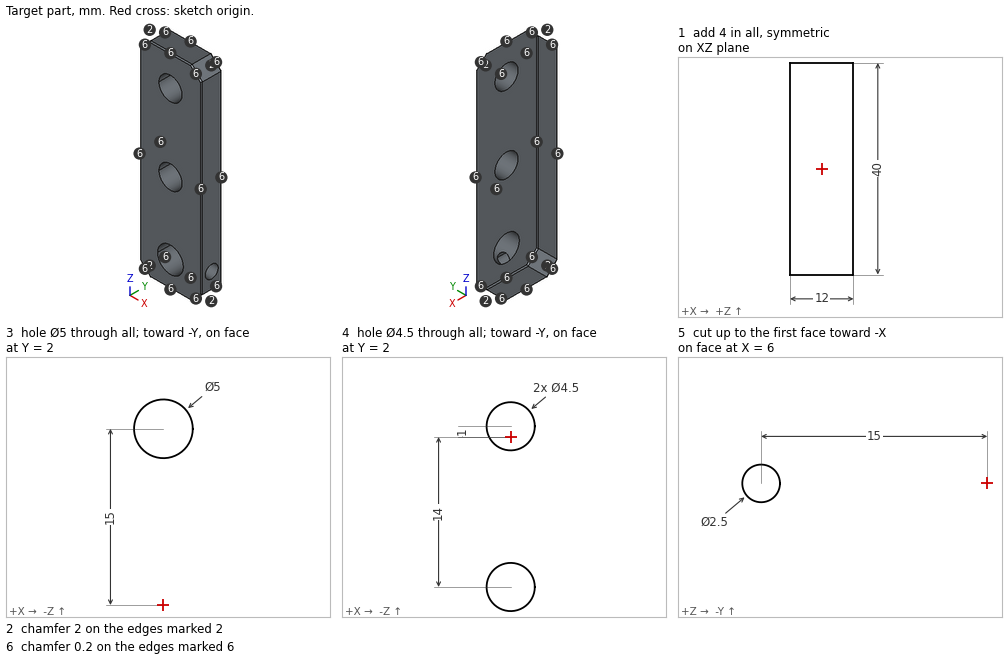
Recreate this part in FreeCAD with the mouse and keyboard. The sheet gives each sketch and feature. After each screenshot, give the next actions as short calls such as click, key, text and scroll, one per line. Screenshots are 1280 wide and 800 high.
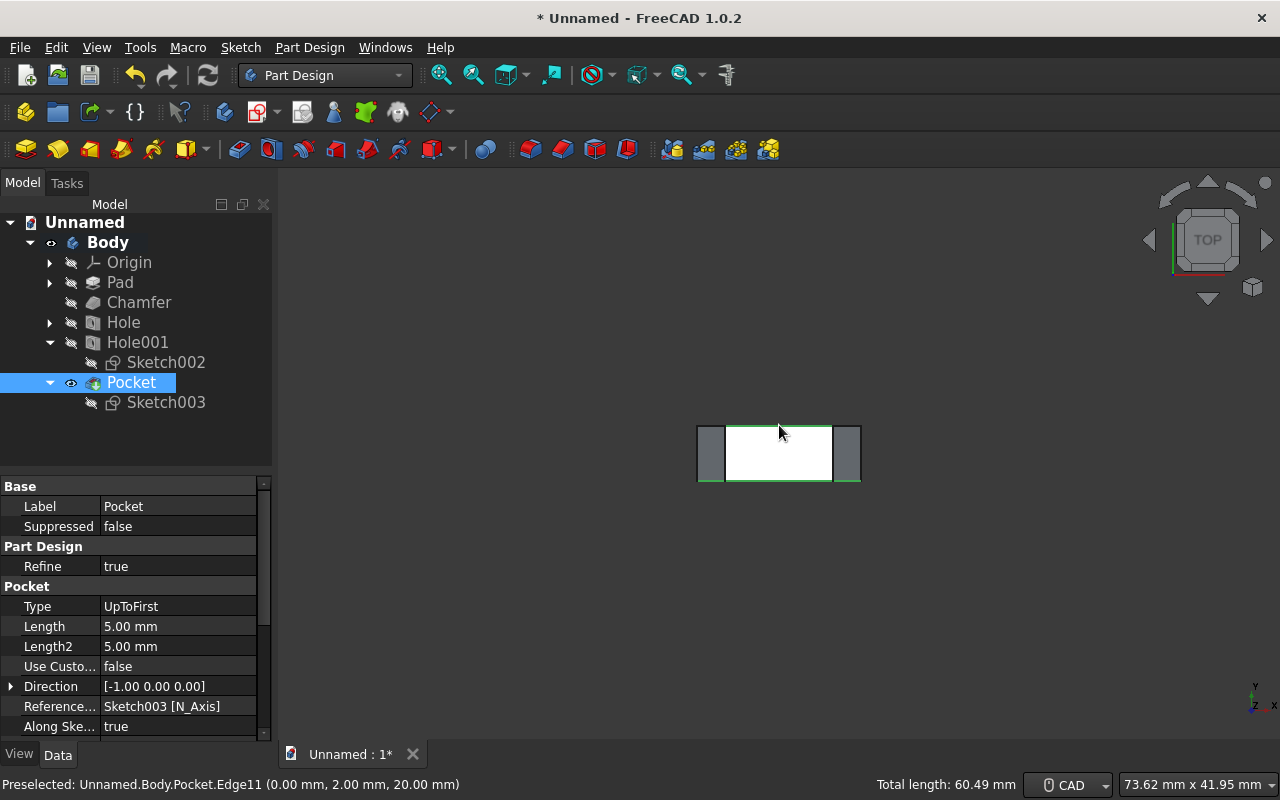
click(711, 425, ctrl)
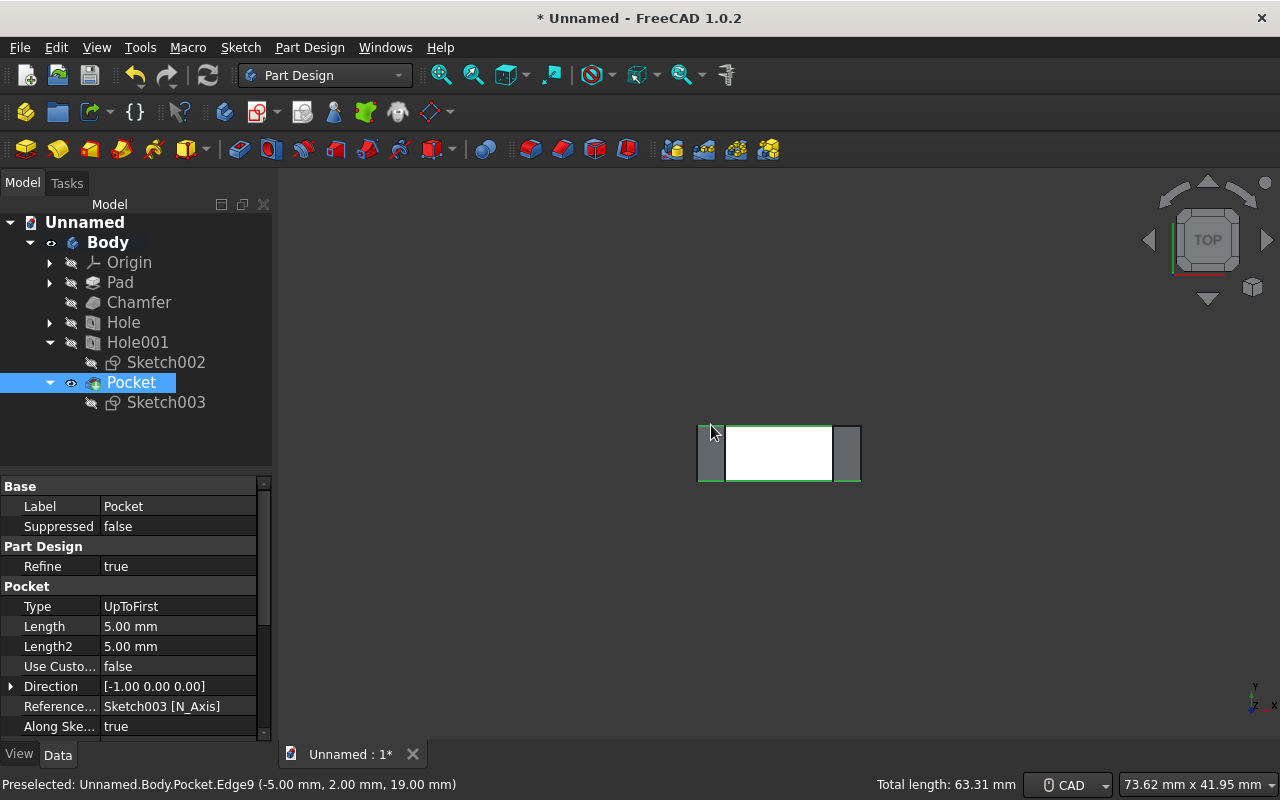
click(847, 425, ctrl)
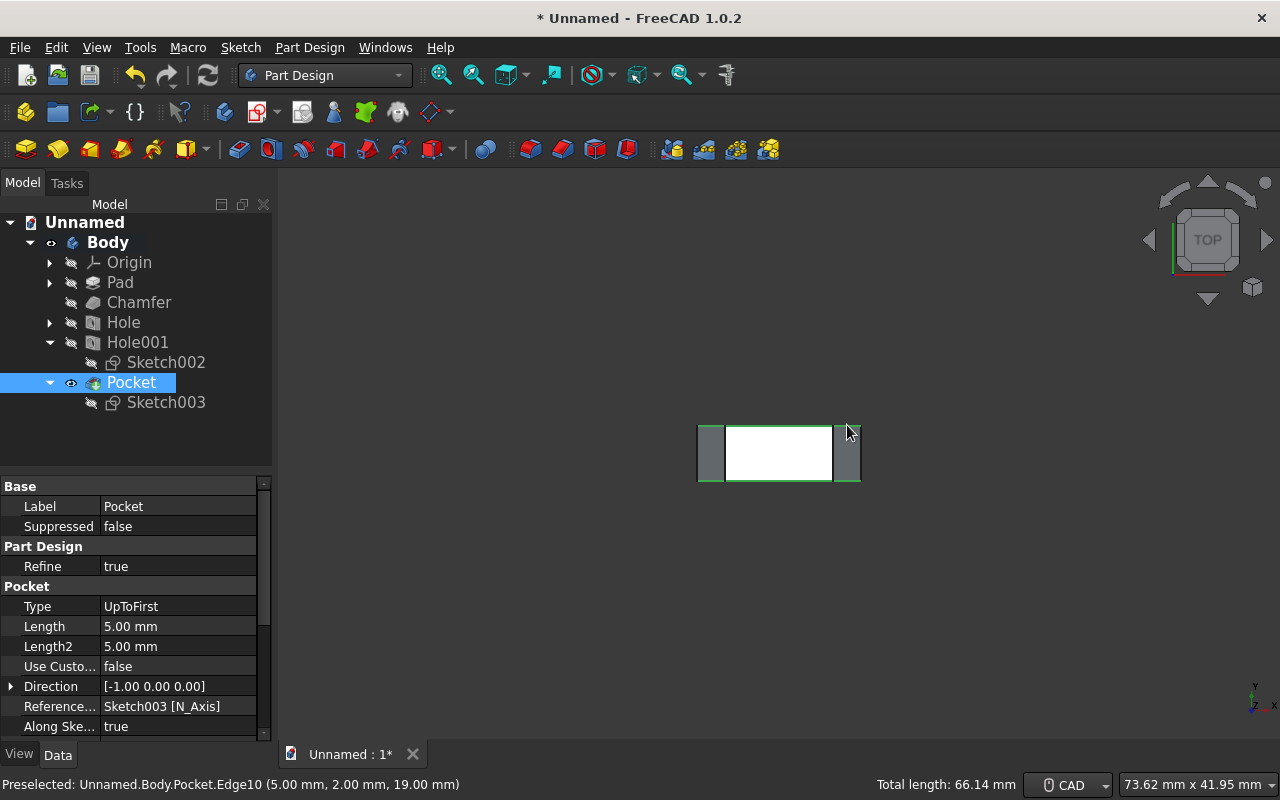
key(0)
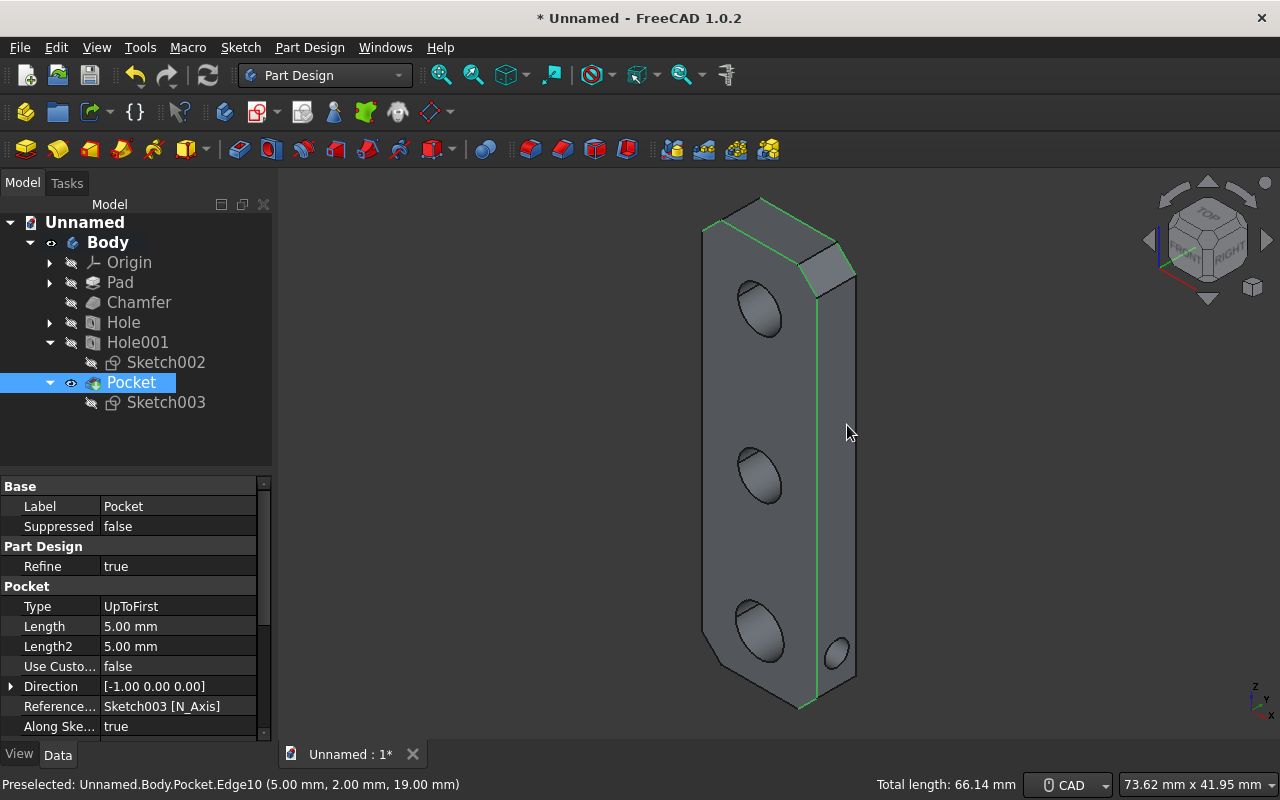
key(1)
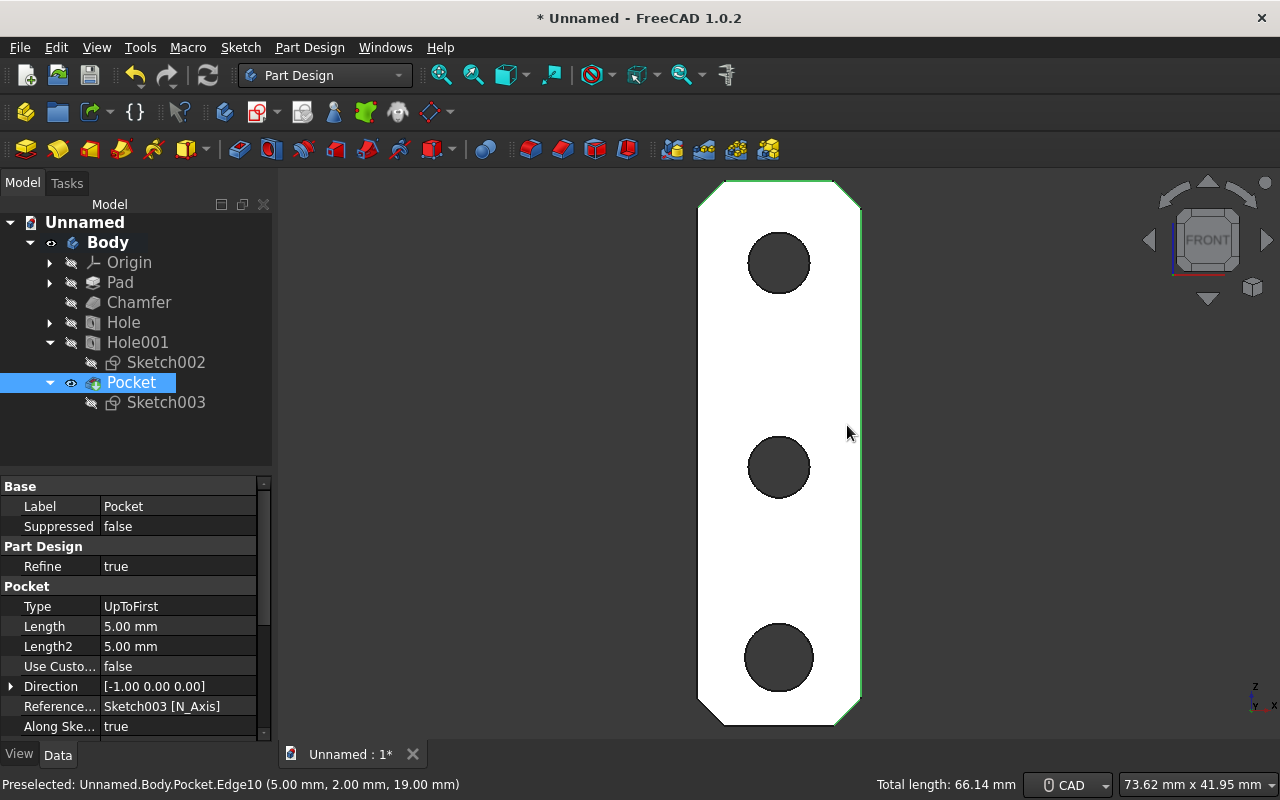
click(697, 452, ctrl)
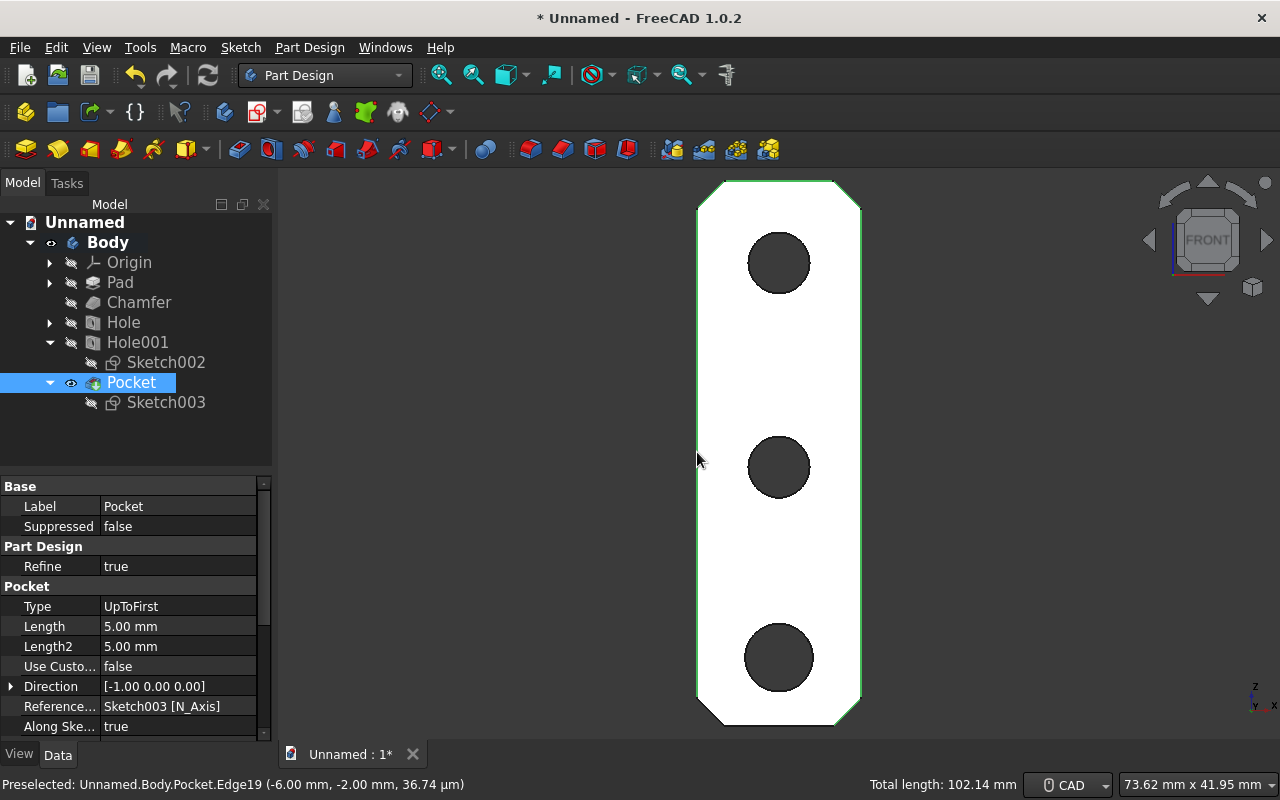
key(3)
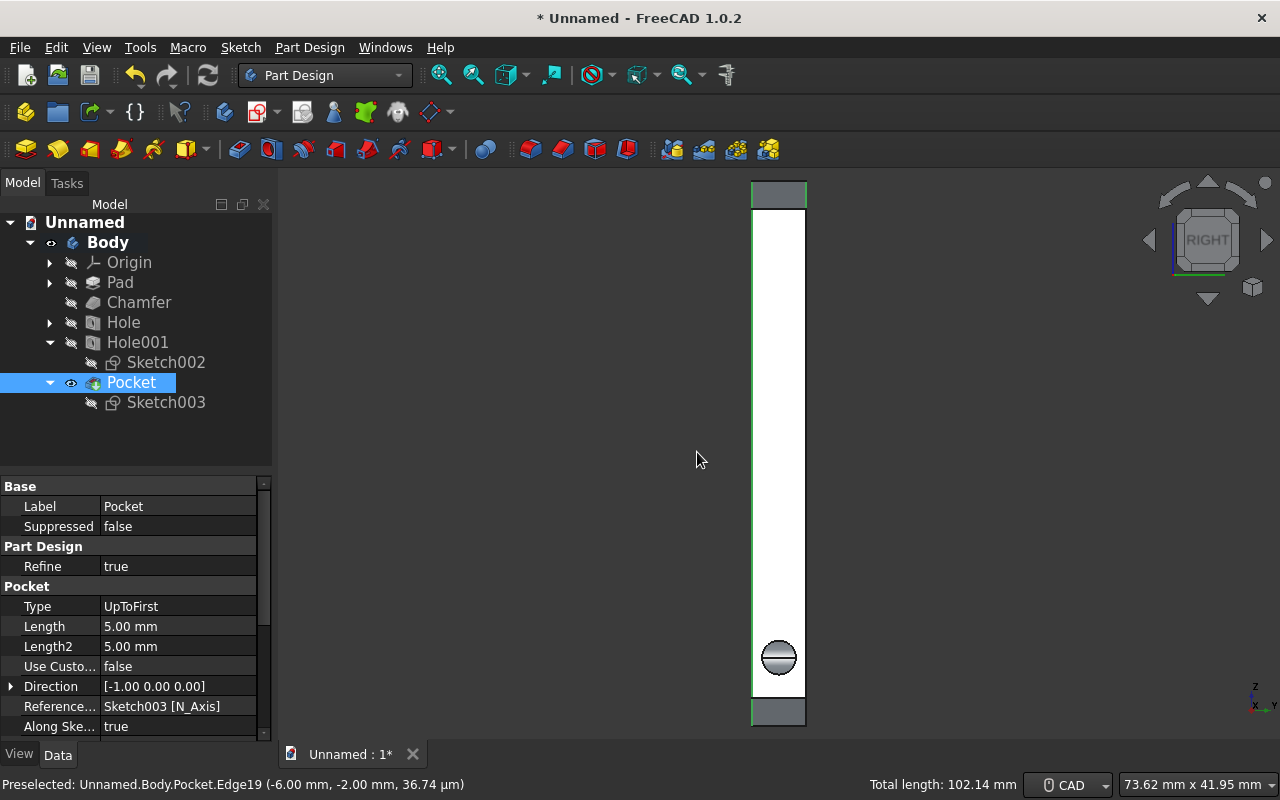
click(806, 452, ctrl)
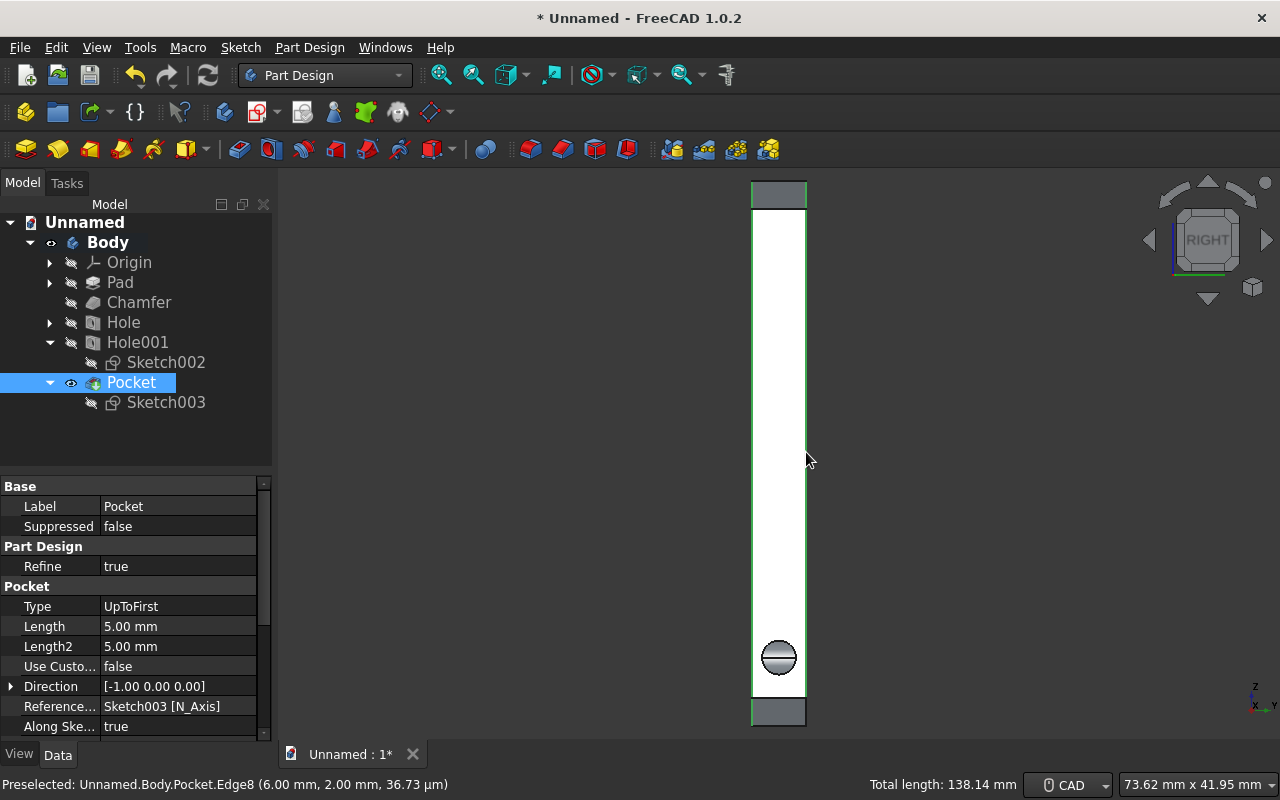
click(806, 708, ctrl)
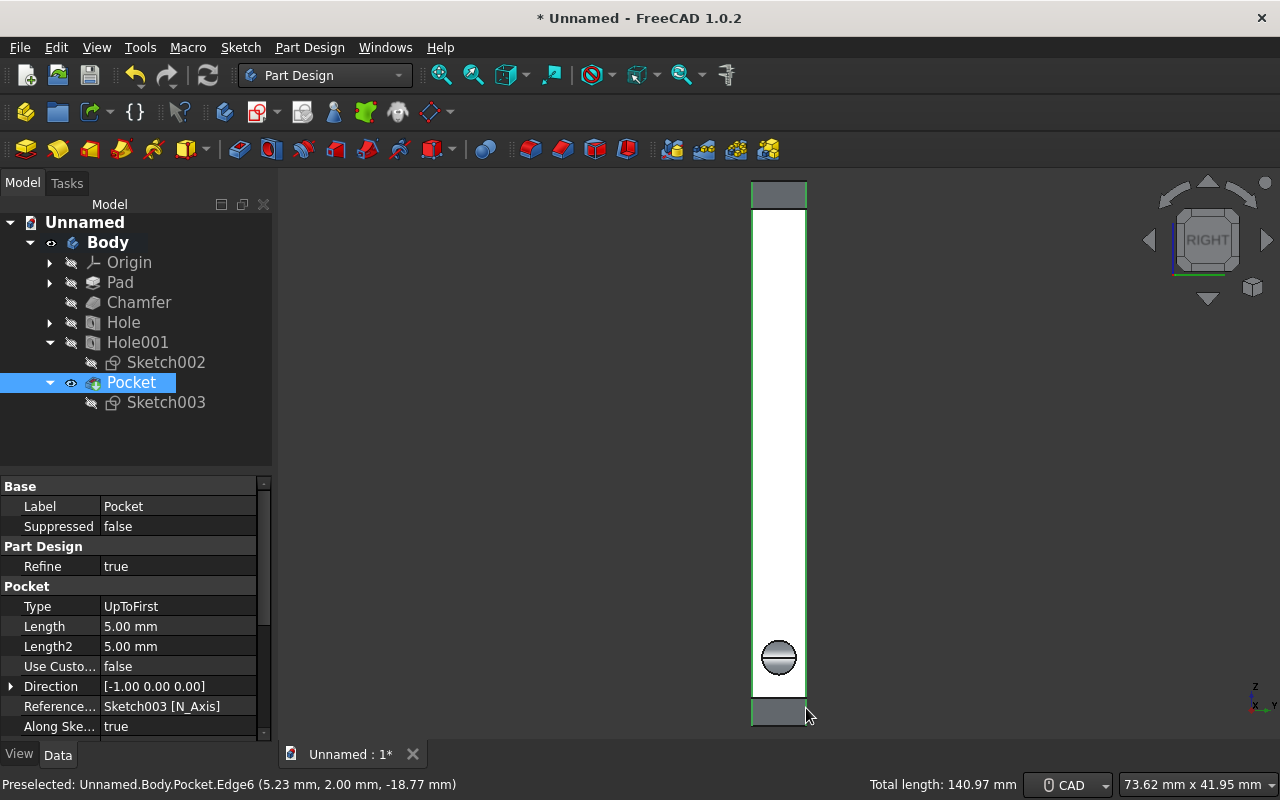
key(5)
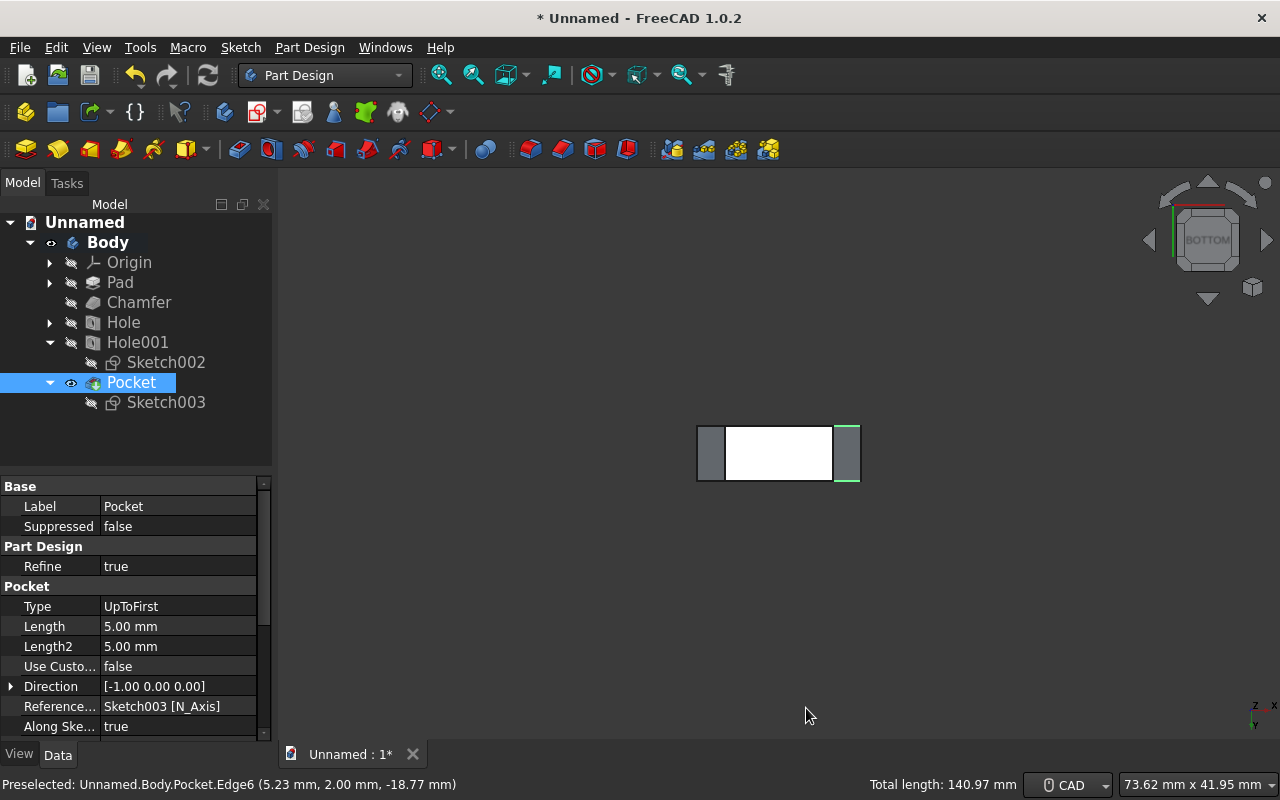
click(442, 76)